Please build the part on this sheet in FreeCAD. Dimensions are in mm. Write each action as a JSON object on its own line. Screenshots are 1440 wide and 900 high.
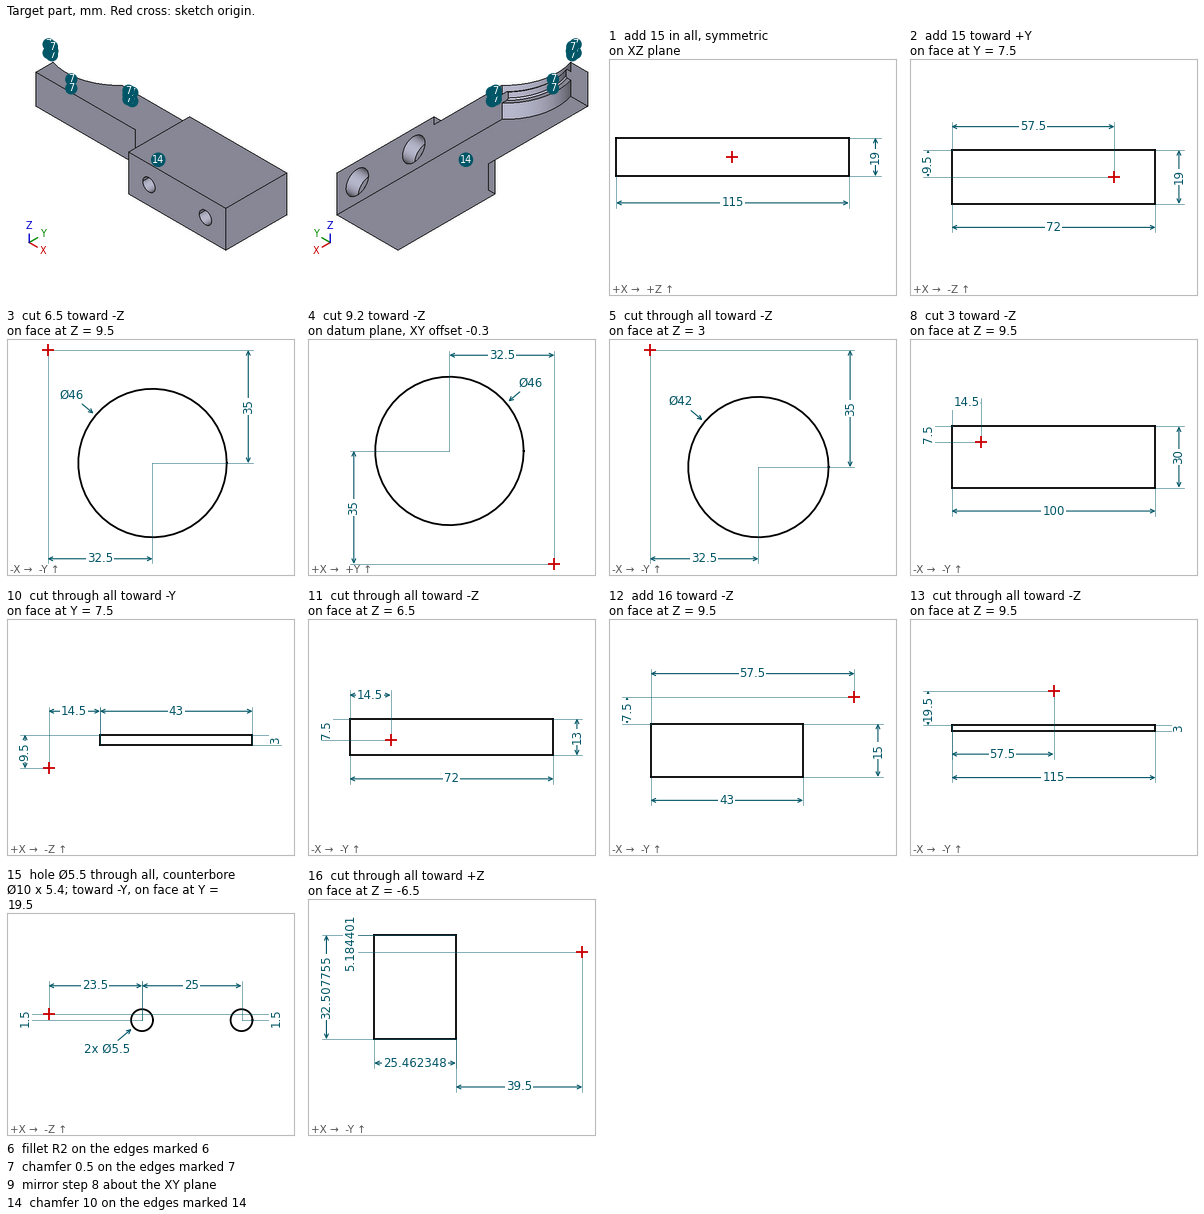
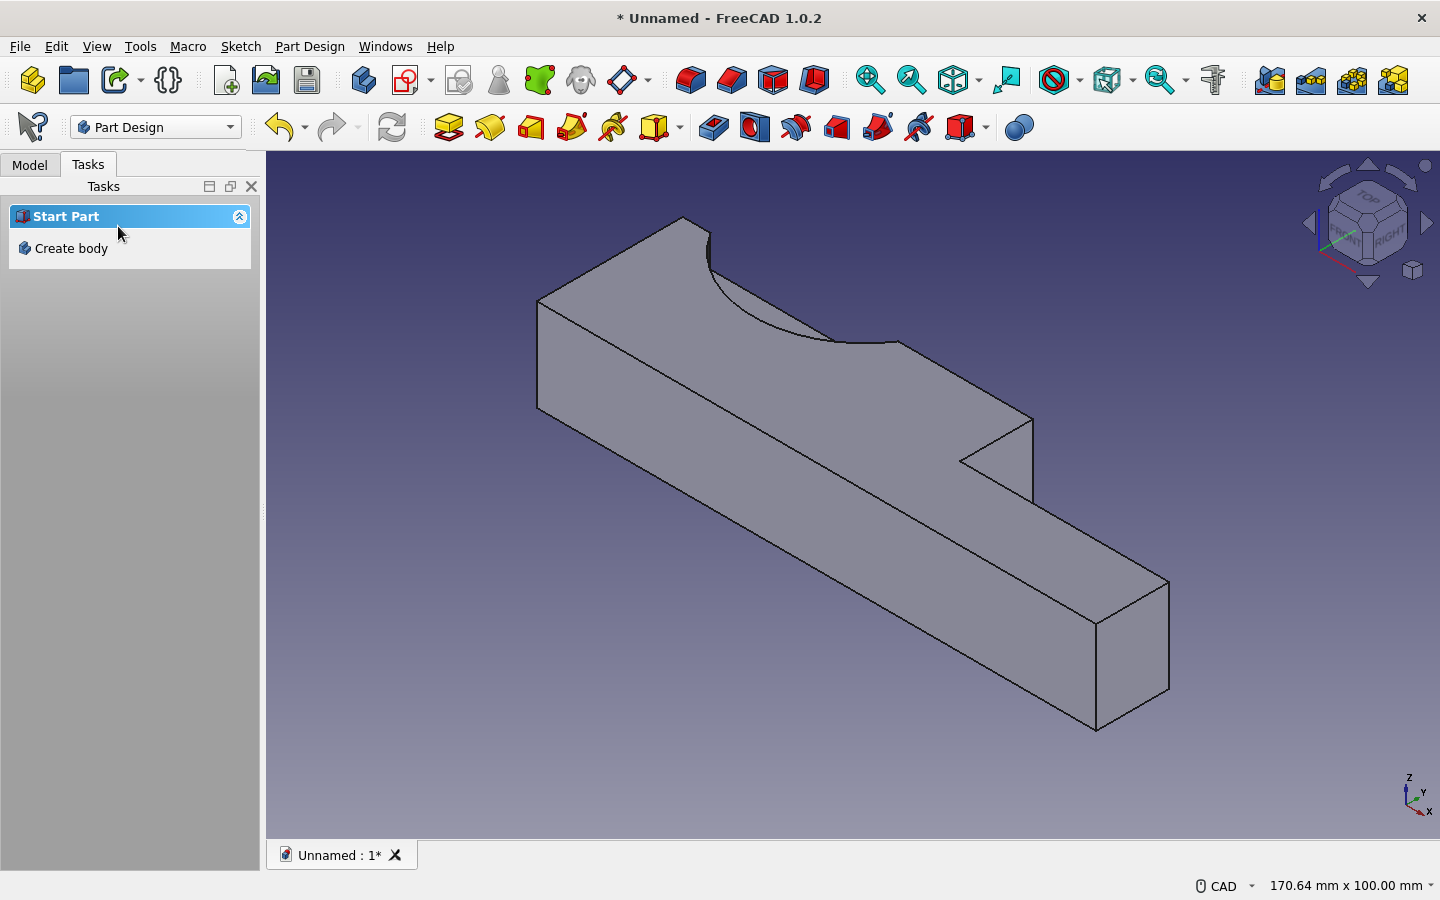
{"action": "left_click", "coordinate": [30, 164]}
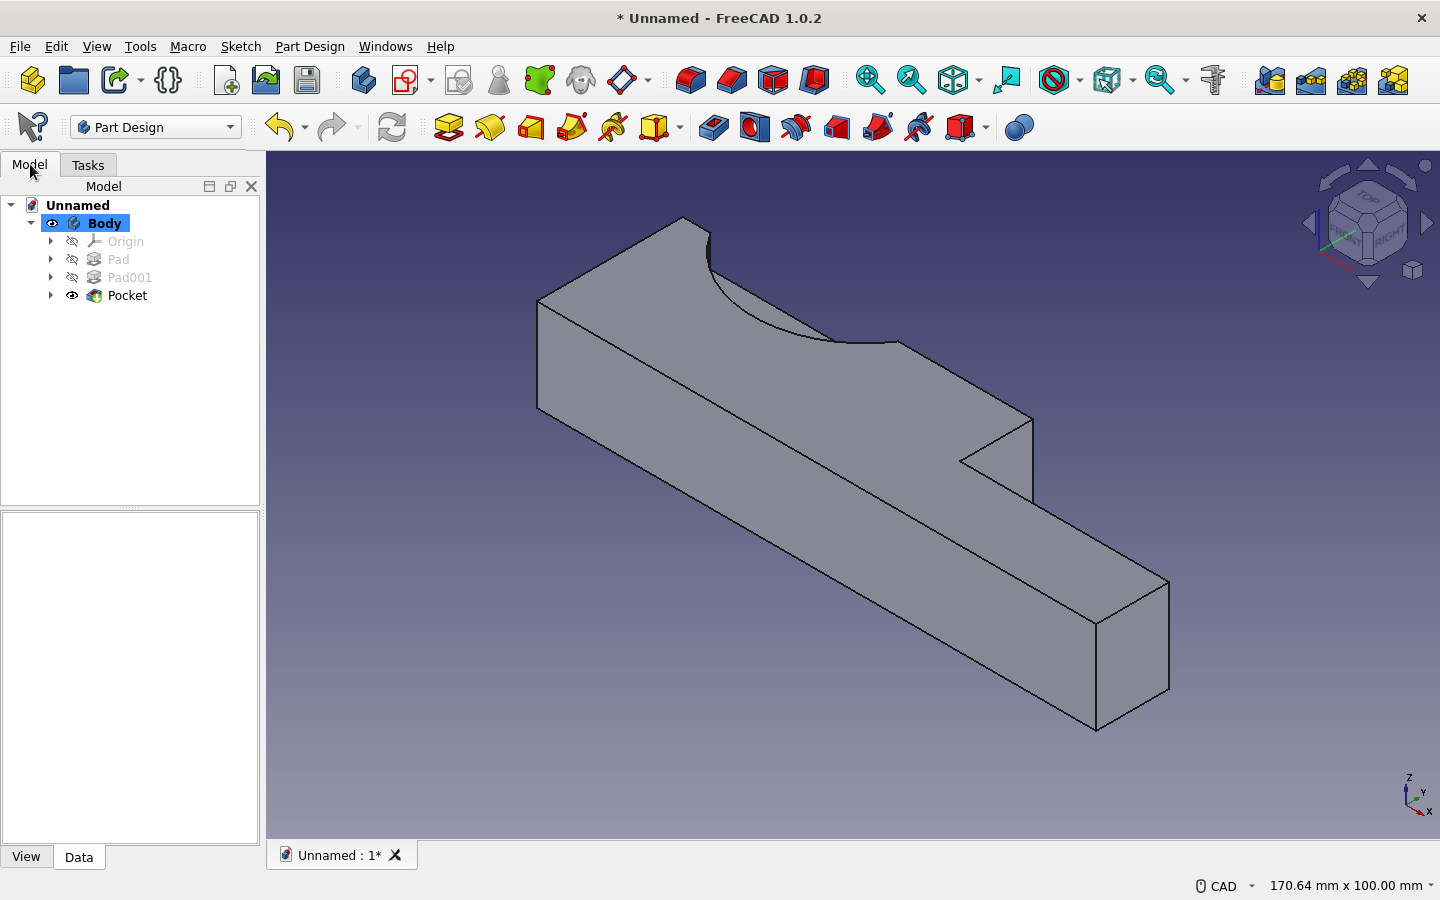
{"action": "left_click", "coordinate": [51, 241]}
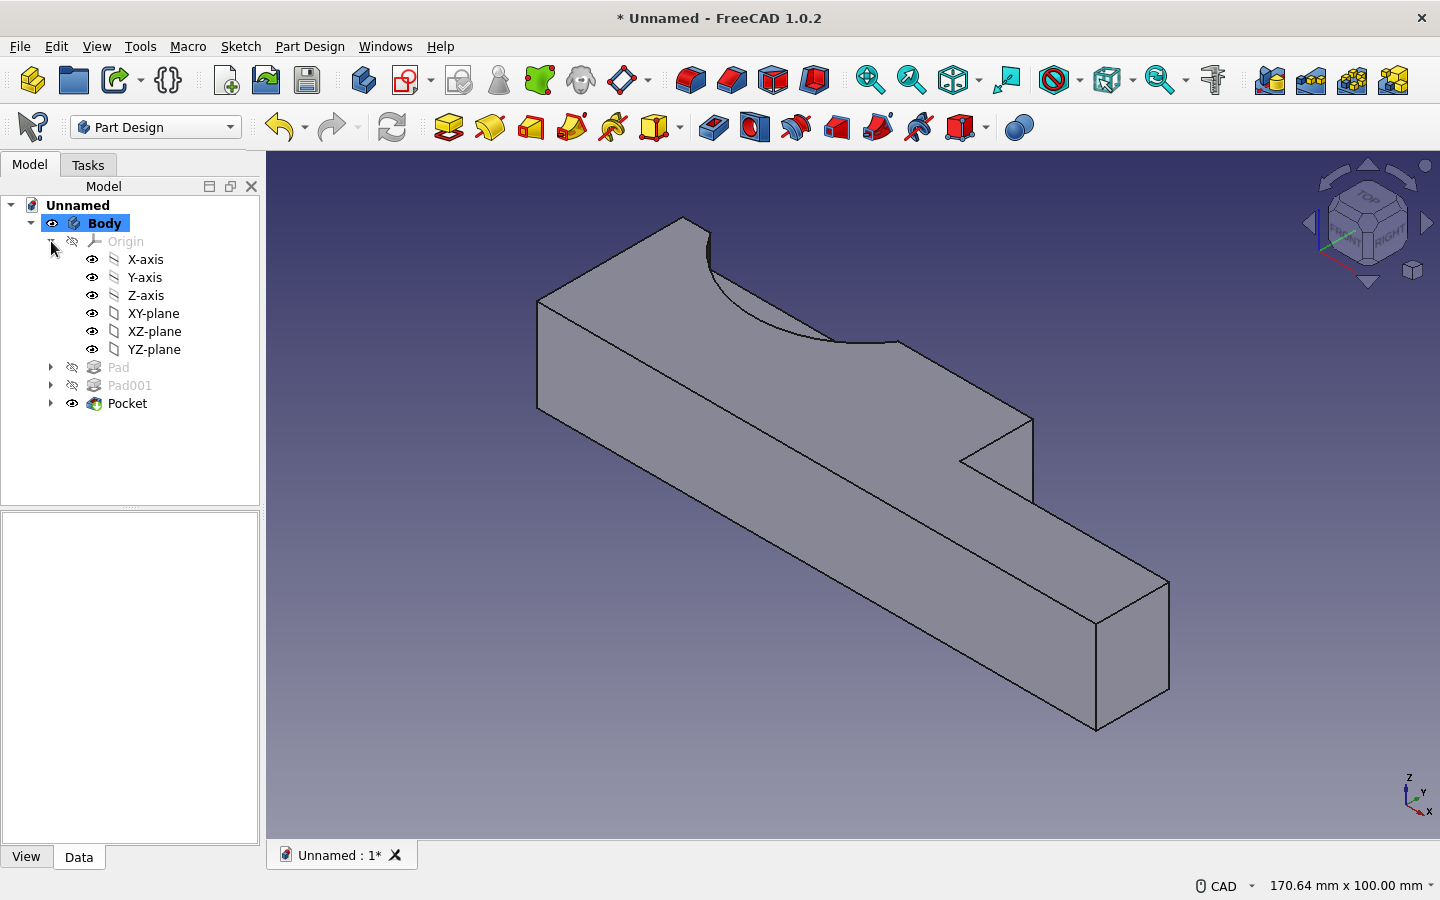
{"action": "left_click", "coordinate": [137, 313]}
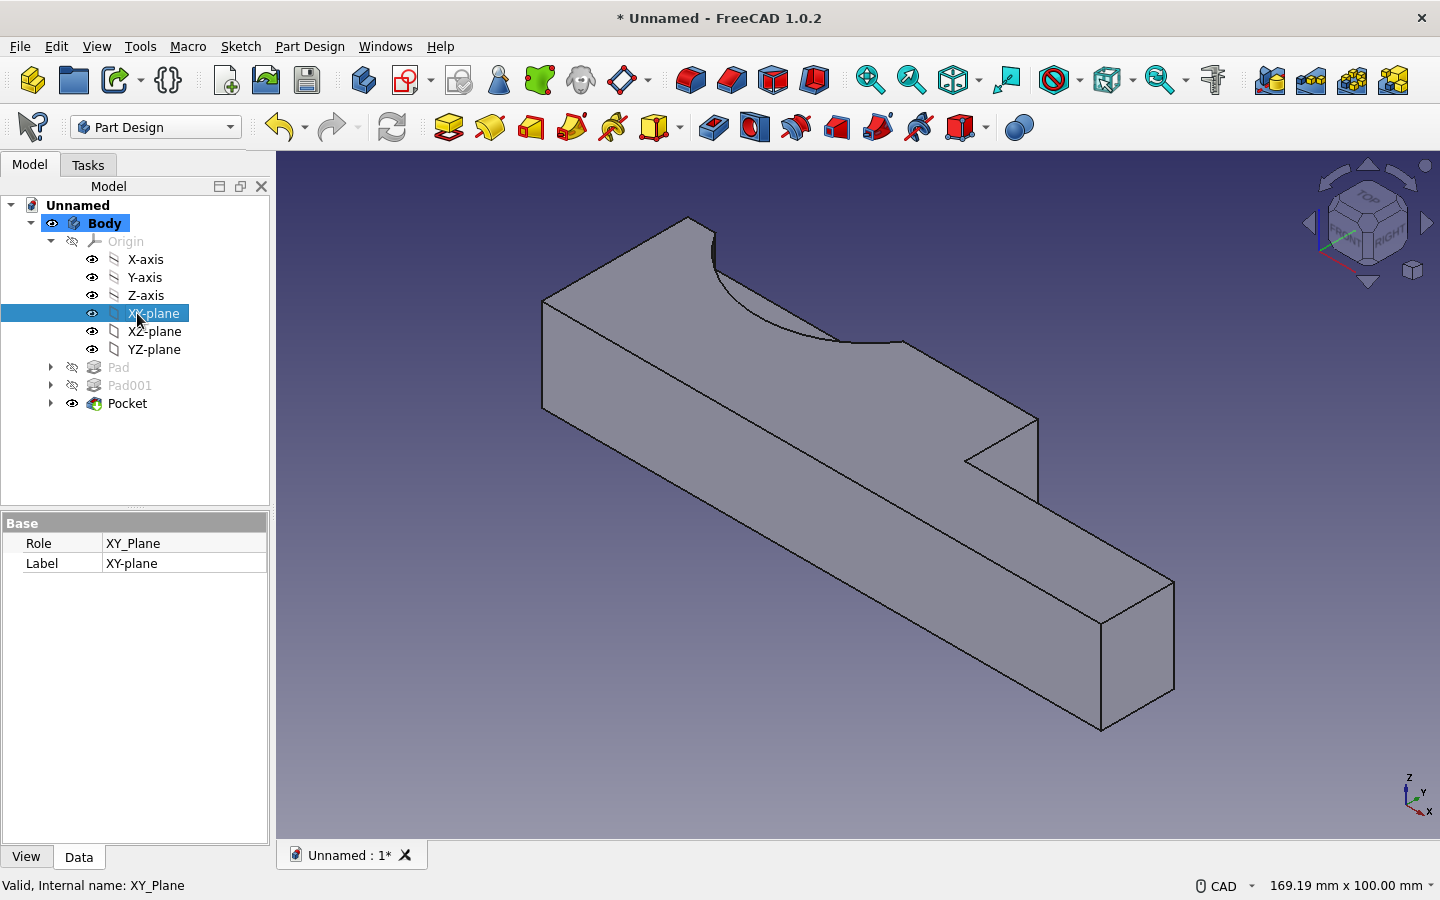
{"action": "left_click", "coordinate": [622, 80]}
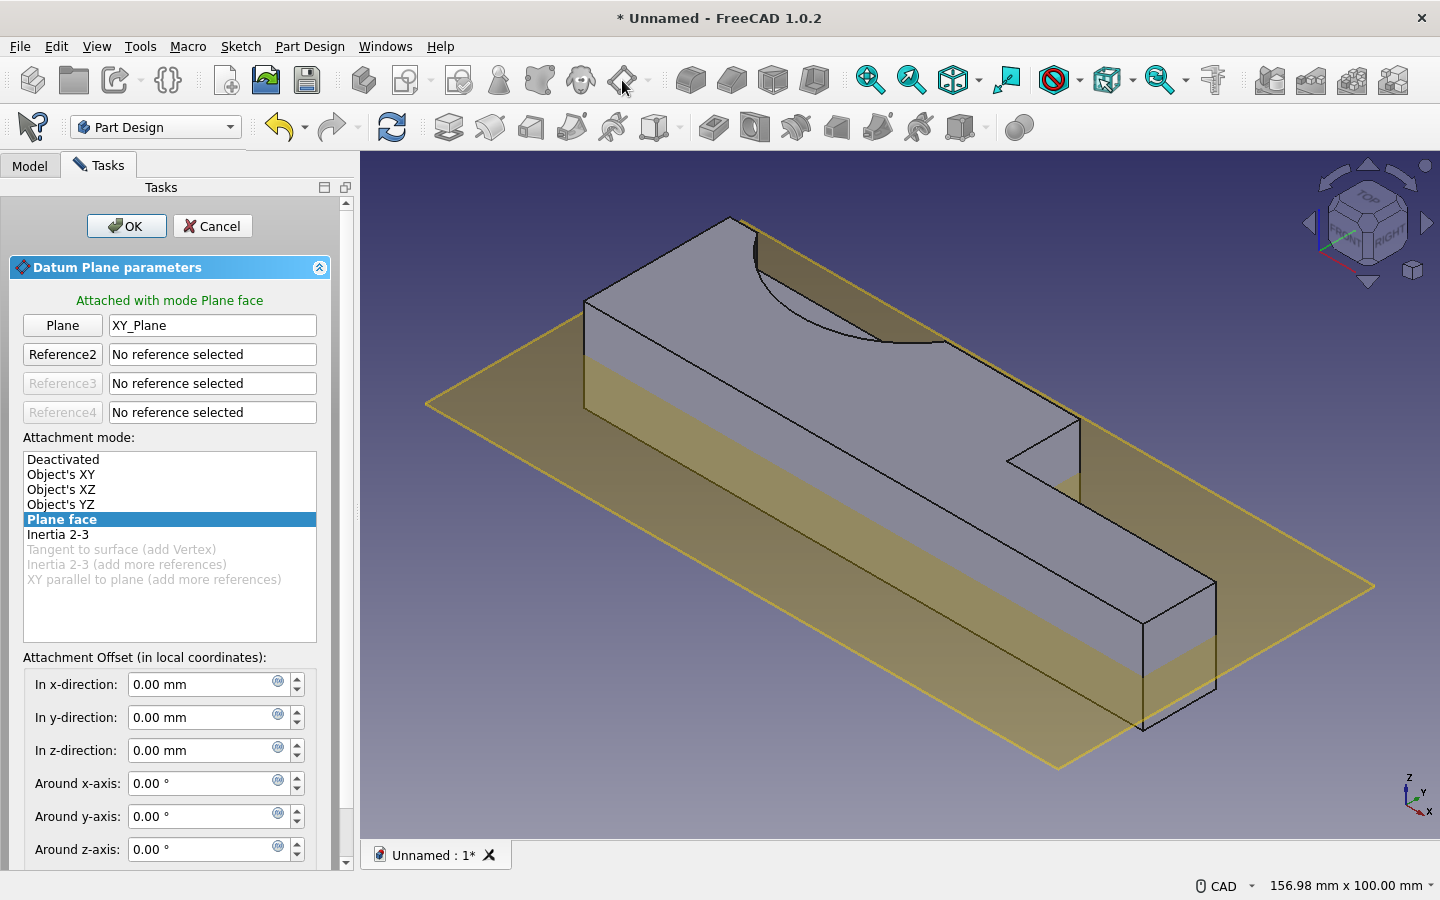
{"action": "triple_click", "coordinate": [210, 750]}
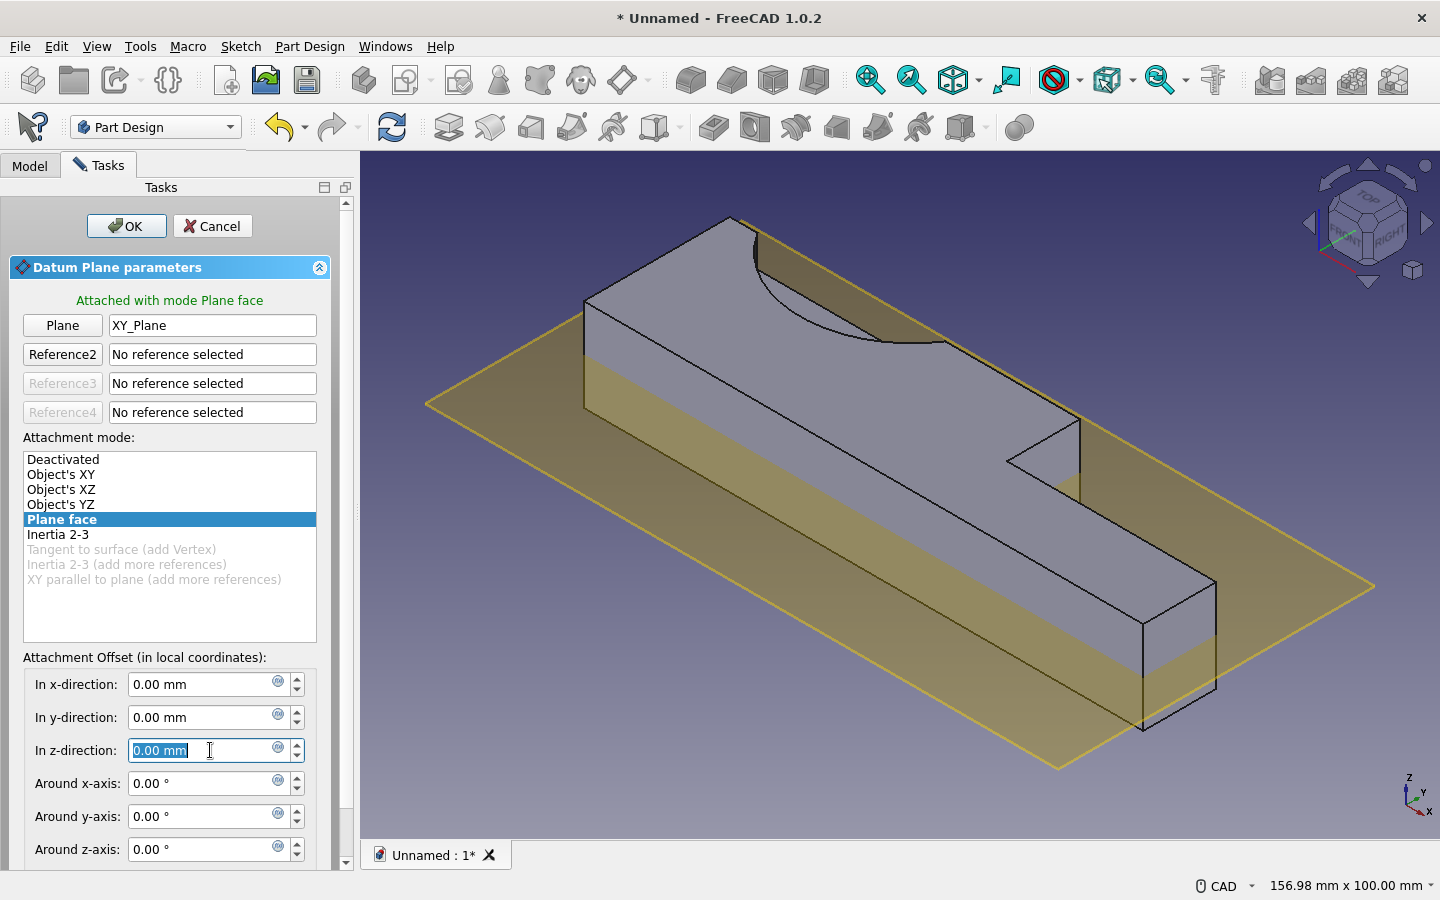
{"action": "type", "text": "-0.3"}
{"action": "key", "text": "Tab"}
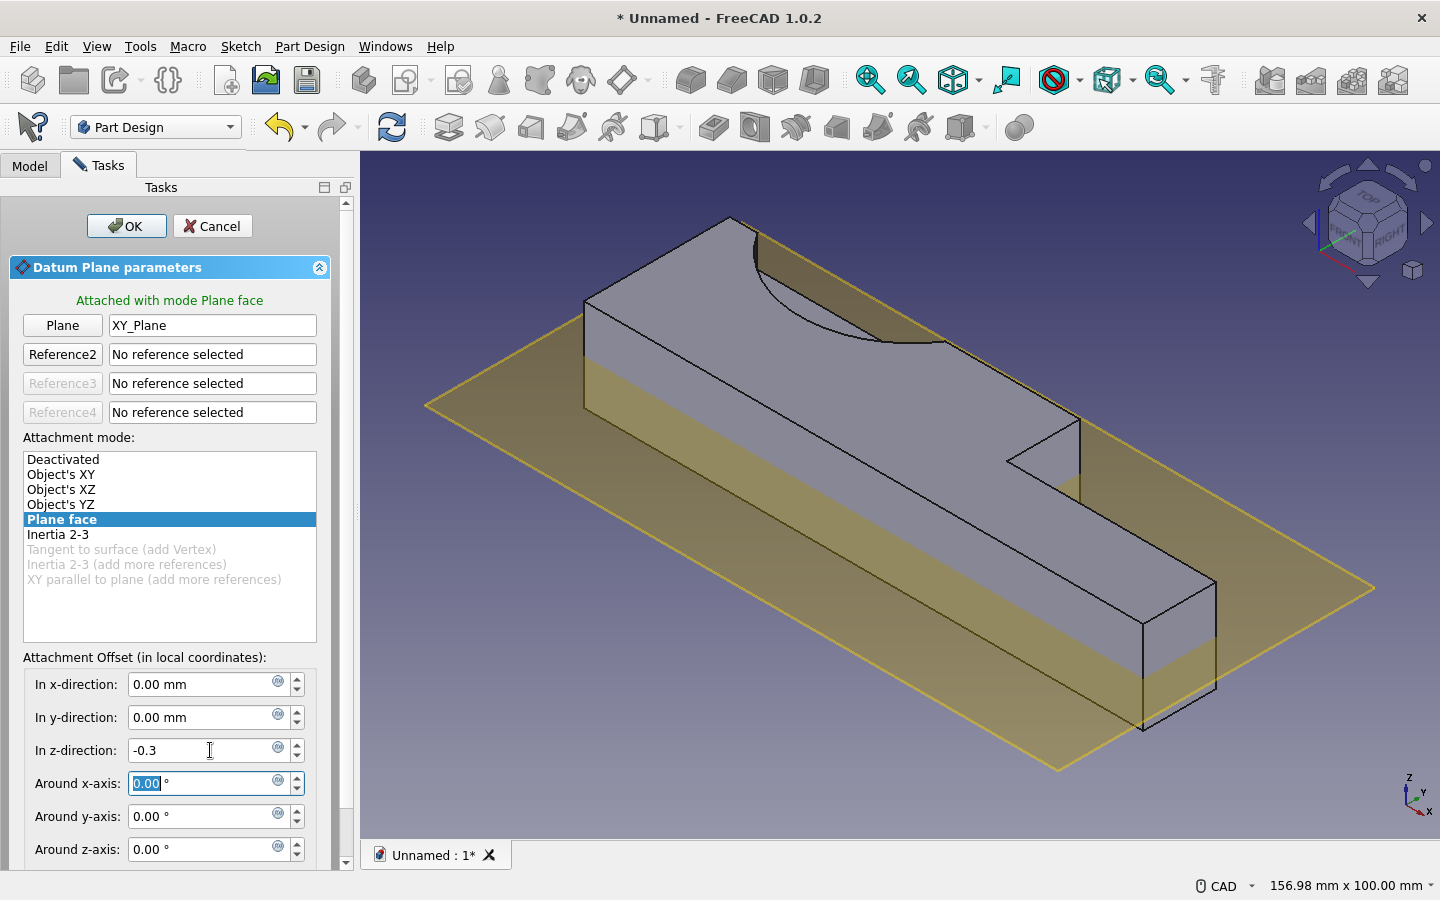
{"action": "left_click", "coordinate": [127, 226]}